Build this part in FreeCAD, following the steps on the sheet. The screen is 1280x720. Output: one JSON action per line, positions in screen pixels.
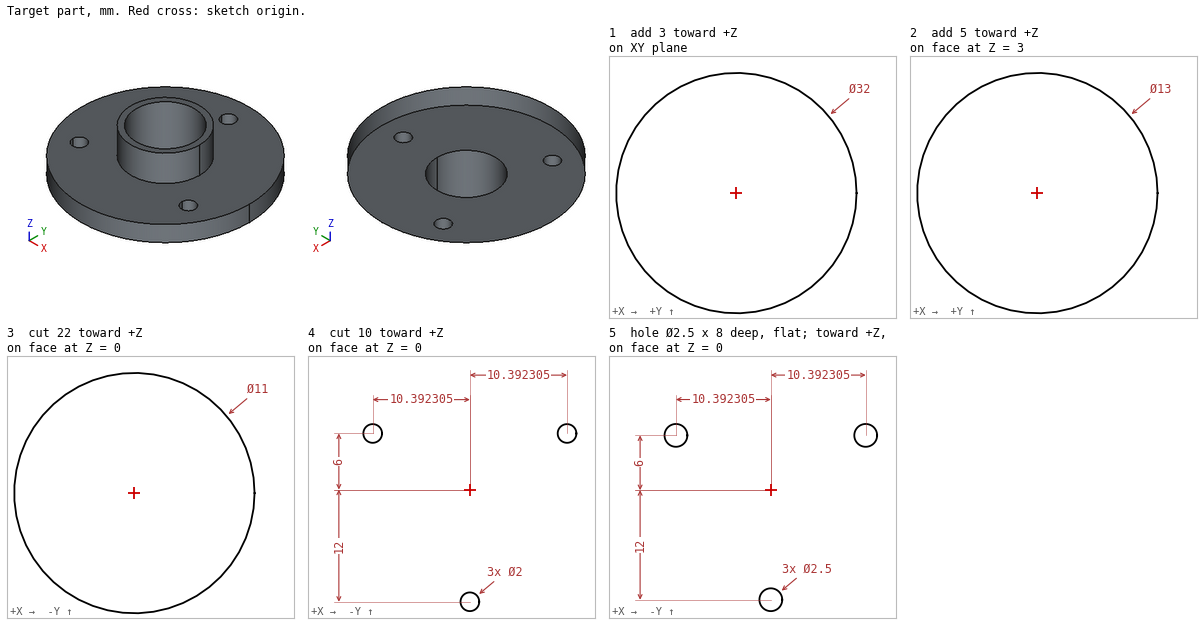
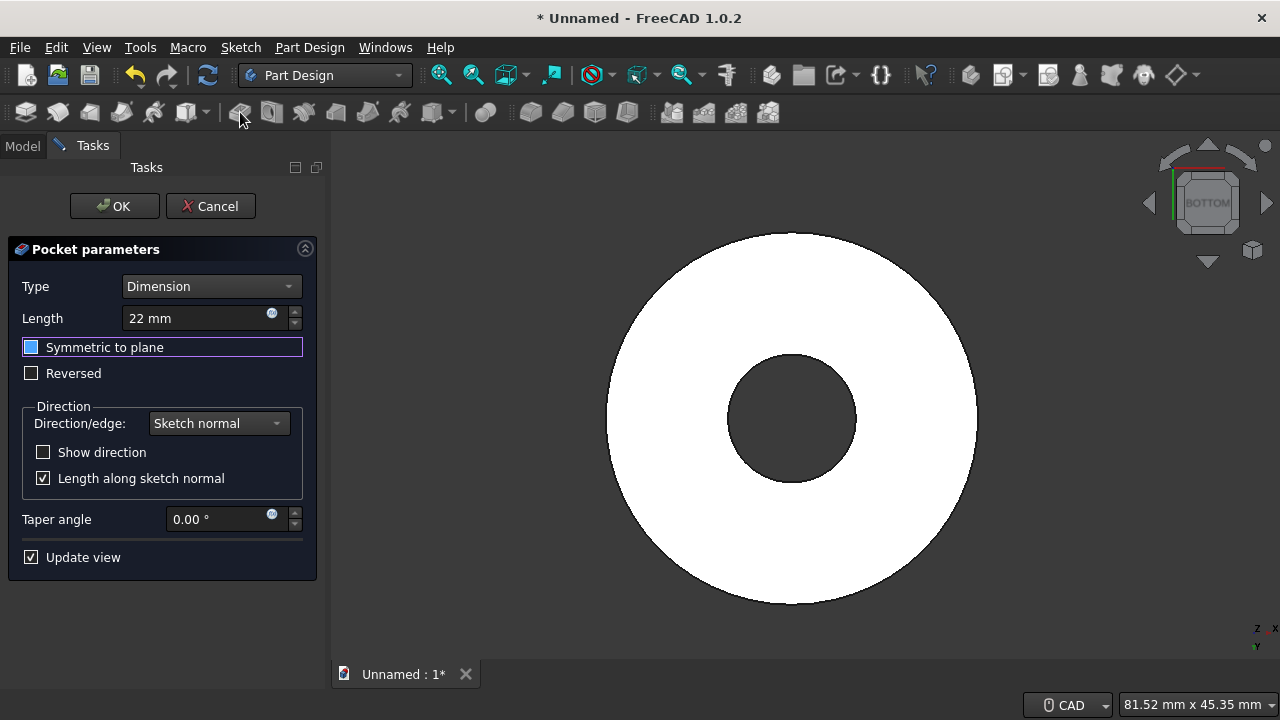
{"action": "left_click", "coordinate": [115, 206]}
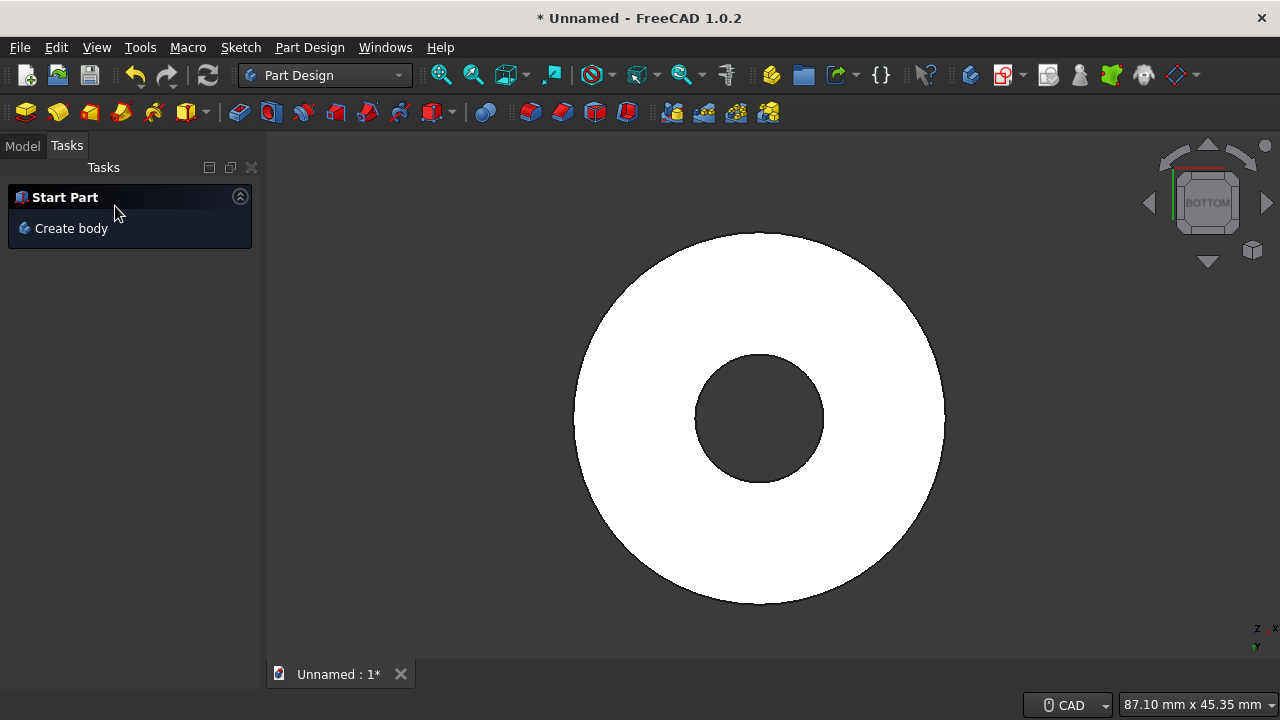
{"action": "left_click", "coordinate": [813, 524]}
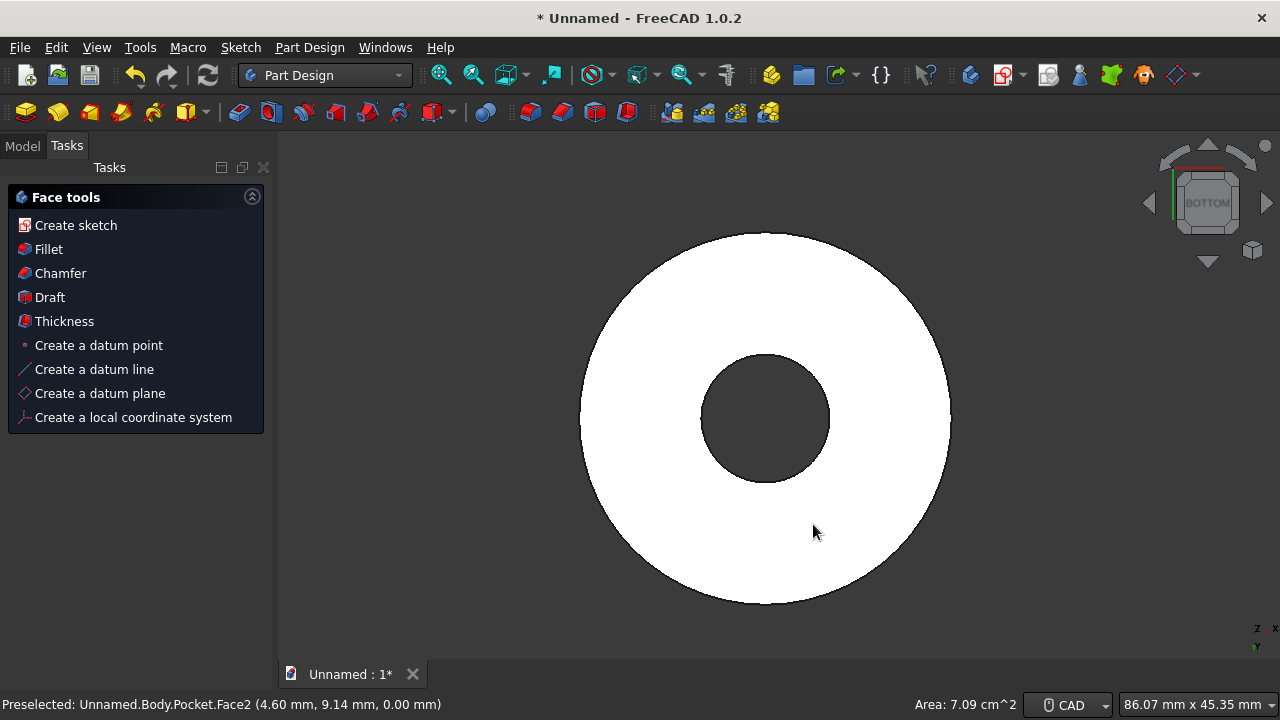
{"action": "left_click", "coordinate": [1004, 76]}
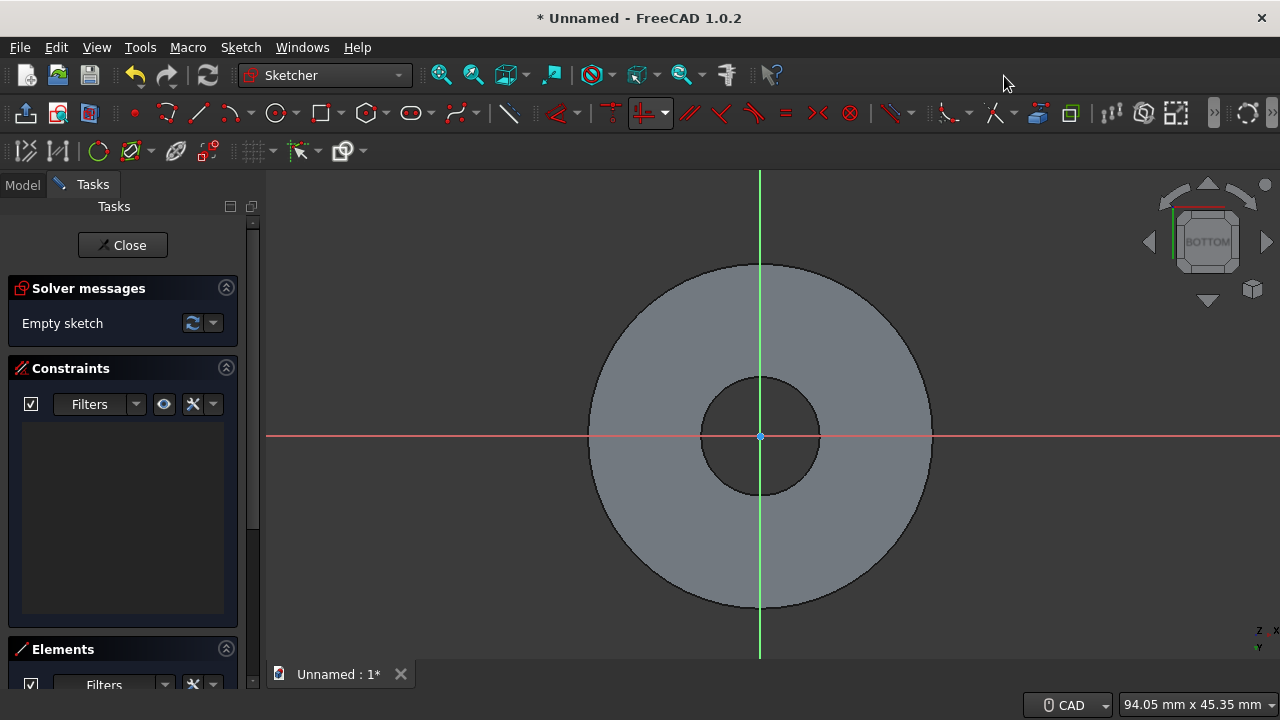
{"action": "scroll", "coordinate": [874, 579], "scroll_direction": "up", "scroll_amount": 2}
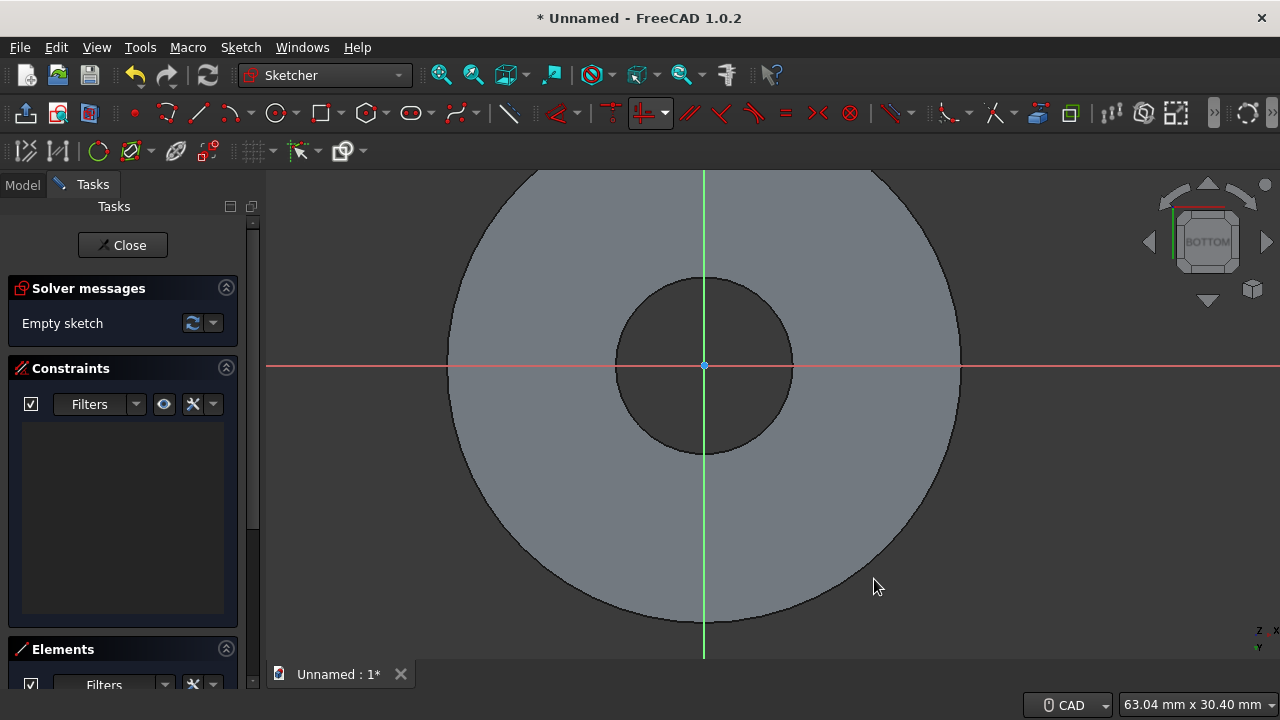
{"action": "left_click", "coordinate": [276, 114]}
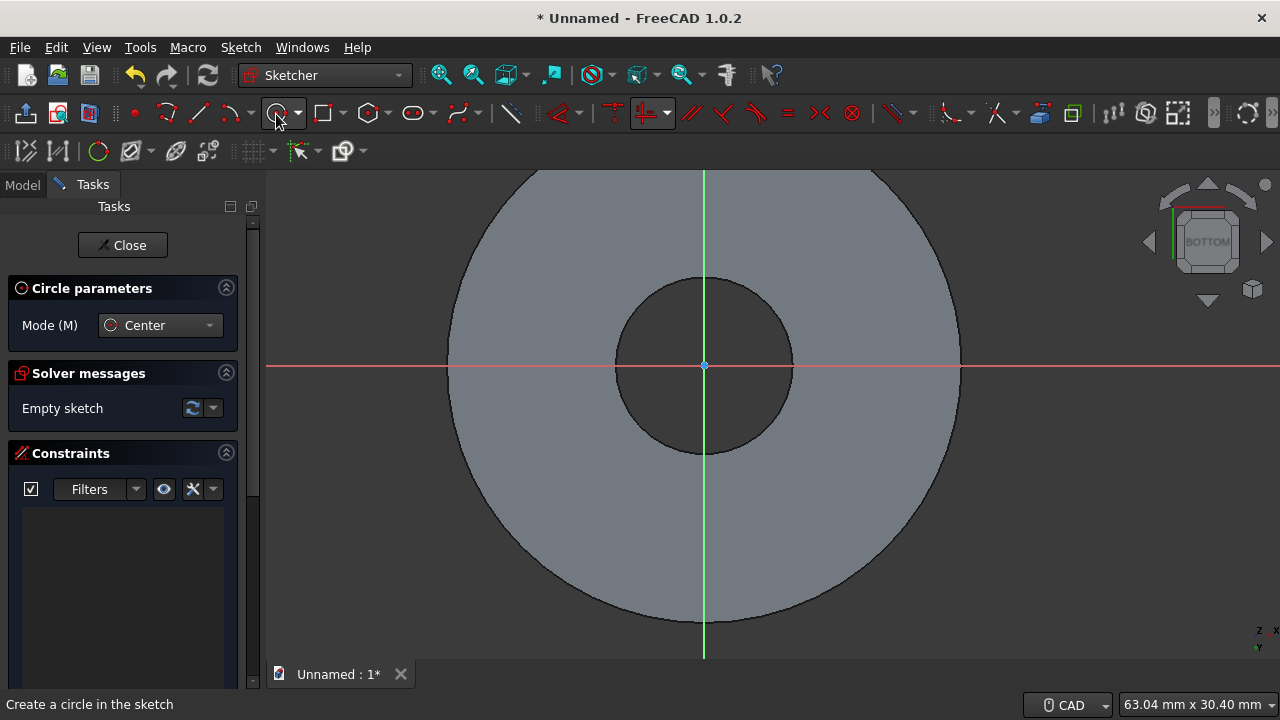
{"action": "scroll", "coordinate": [704, 559], "scroll_direction": "up", "scroll_amount": 2}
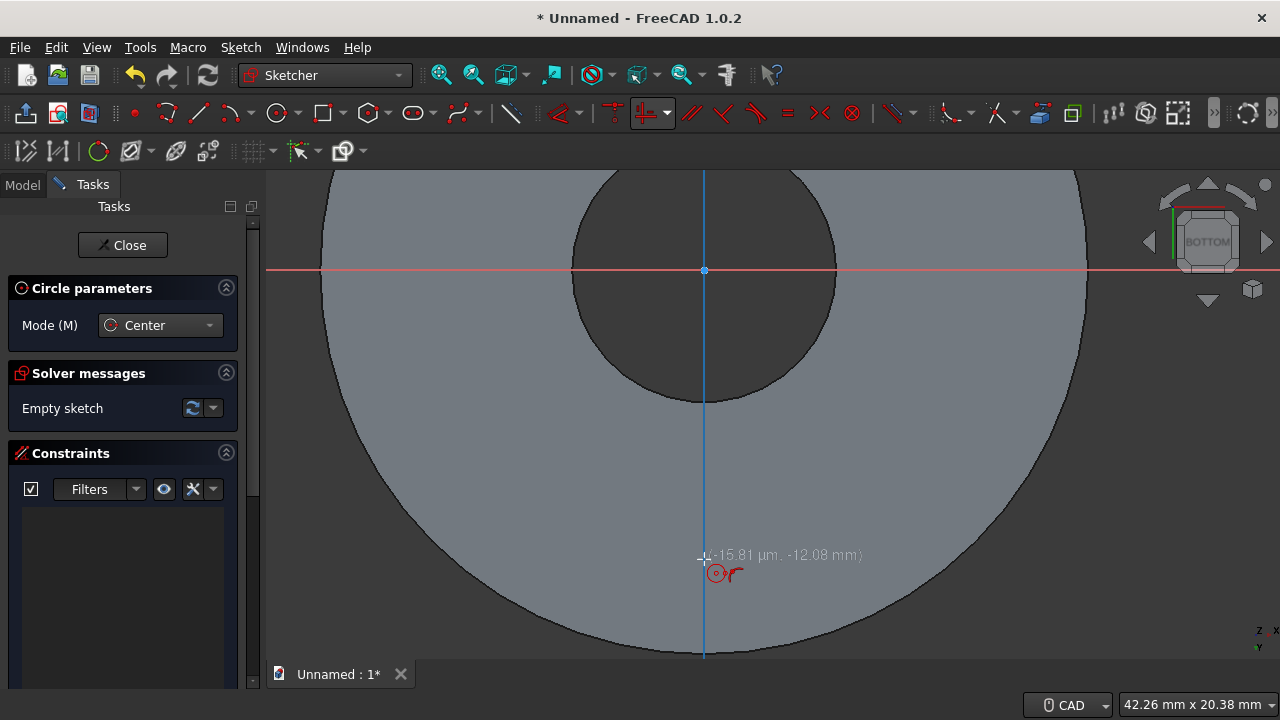
{"action": "left_click", "coordinate": [704, 558]}
{"action": "mouse_move", "coordinate": [721, 541]}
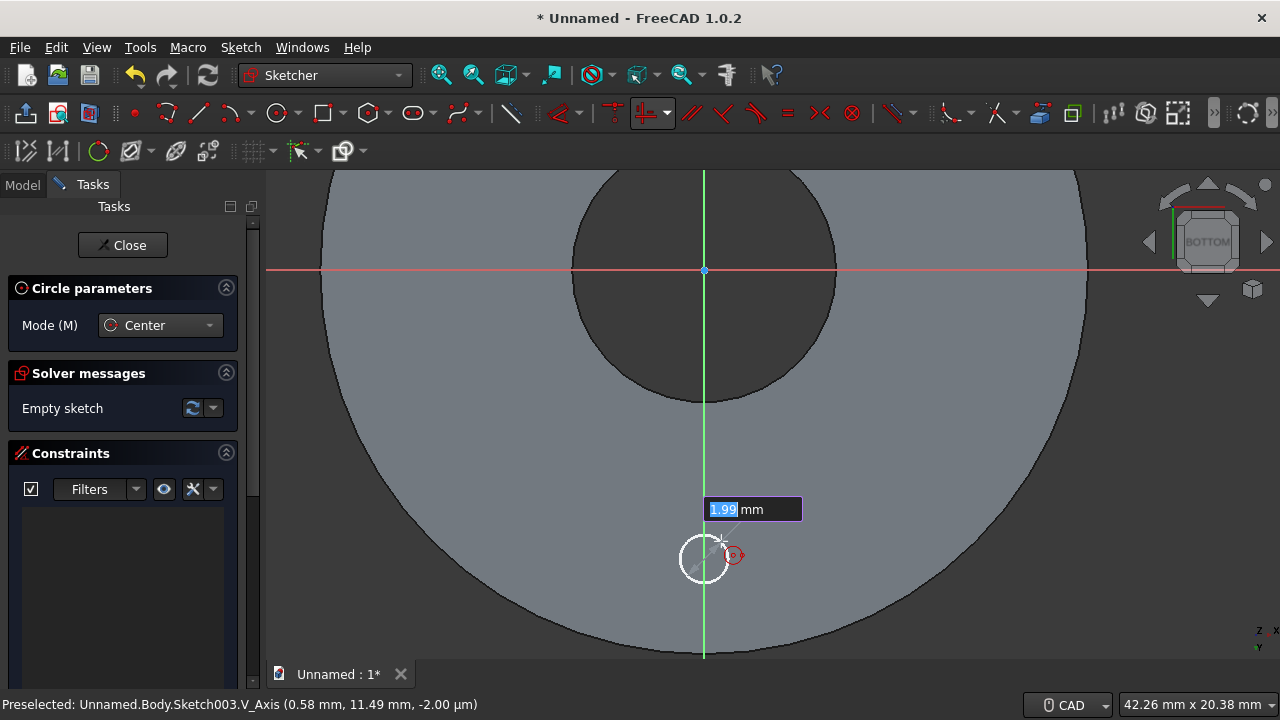
{"action": "type", "text": "2"}
{"action": "key", "text": "Return"}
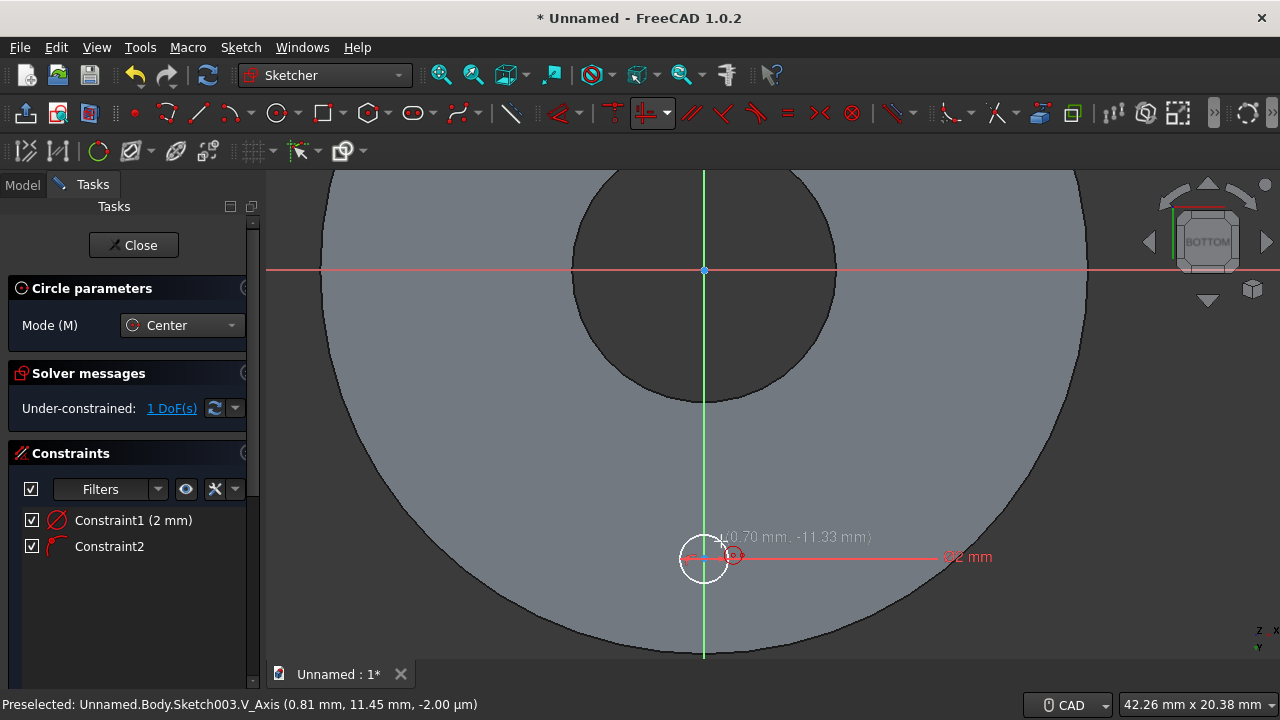
{"action": "scroll", "coordinate": [705, 561], "scroll_direction": "down", "scroll_amount": 2}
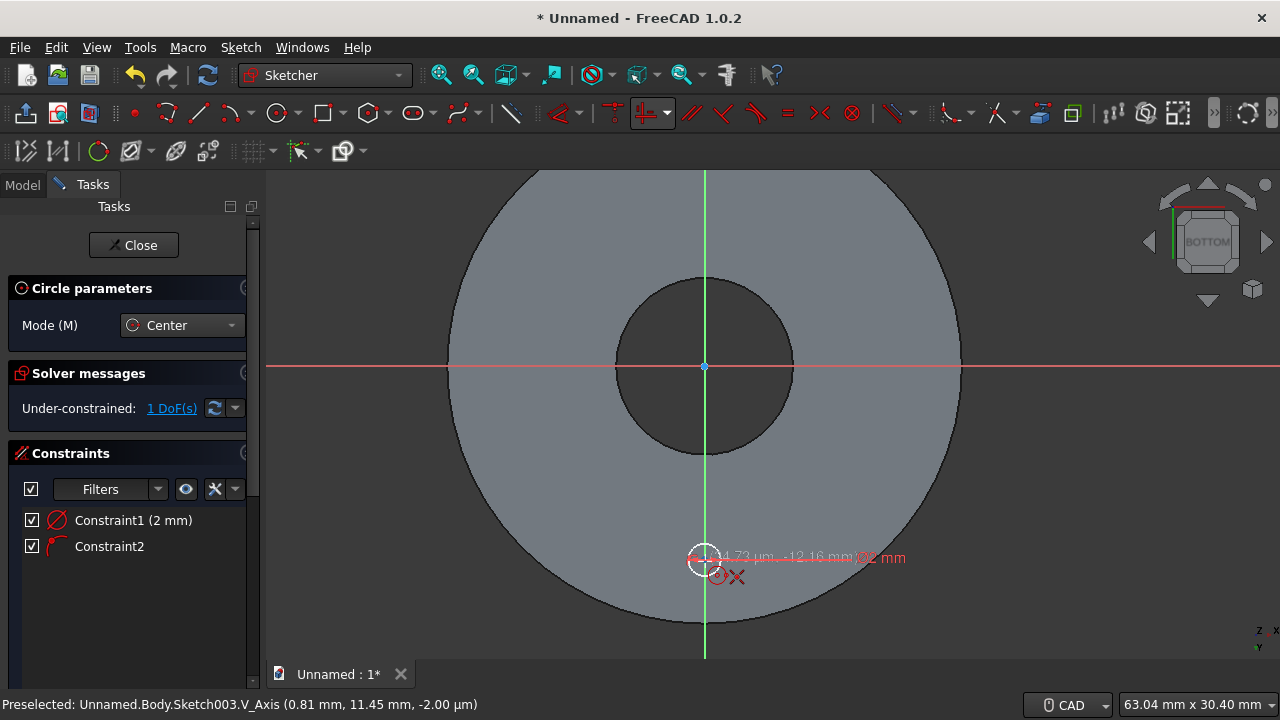
{"action": "scroll", "coordinate": [537, 270], "scroll_direction": "up", "scroll_amount": 2}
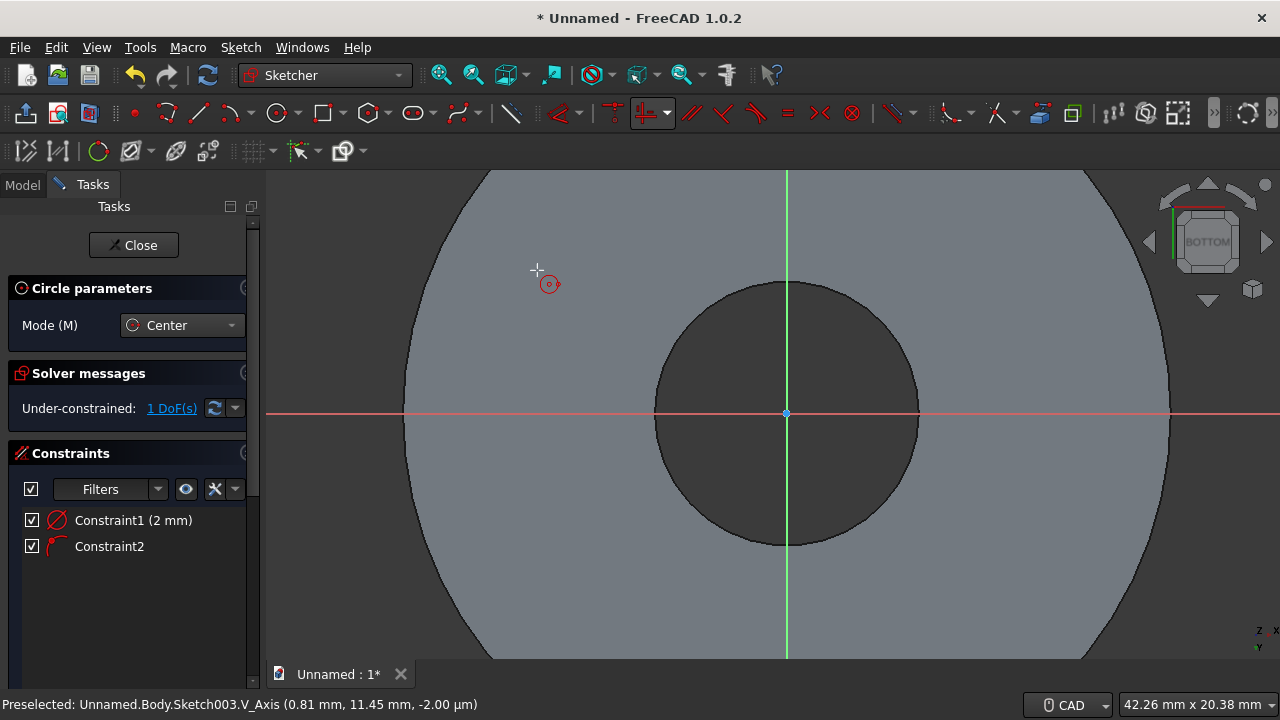
{"action": "left_click", "coordinate": [538, 270]}
{"action": "mouse_move", "coordinate": [554, 253]}